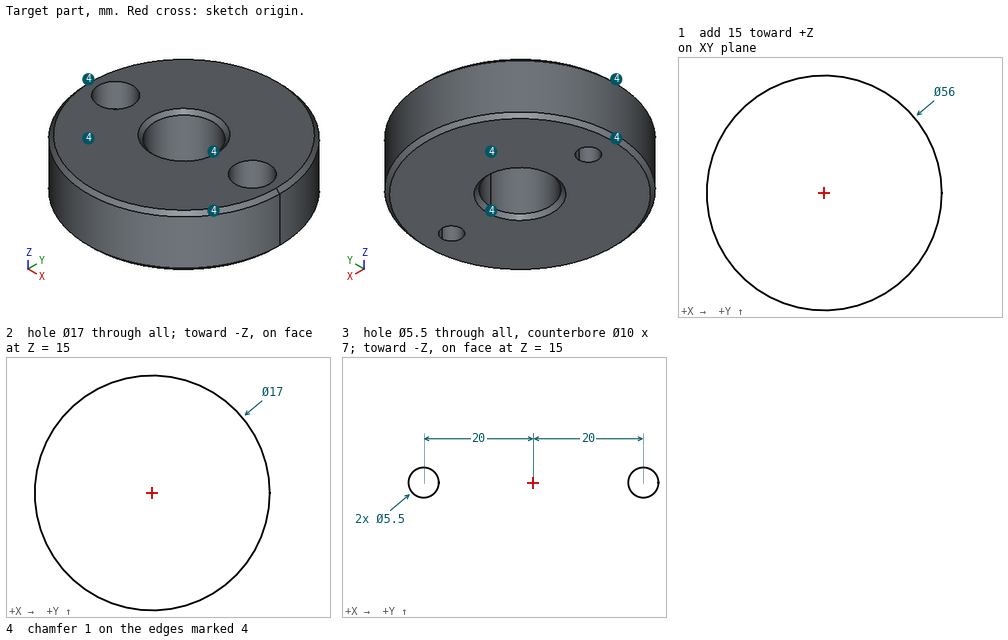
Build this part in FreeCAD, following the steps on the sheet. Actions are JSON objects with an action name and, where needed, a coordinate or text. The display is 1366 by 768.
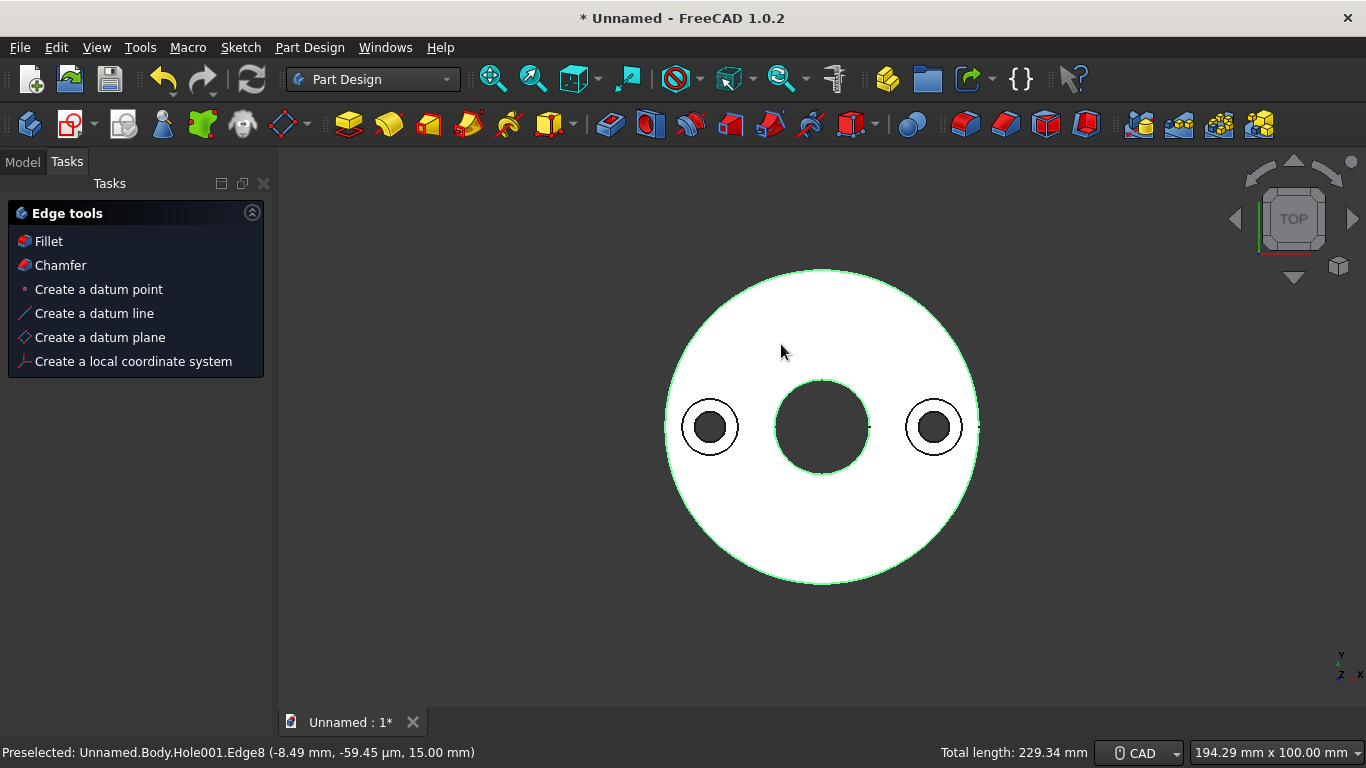
{"action": "key", "text": "1"}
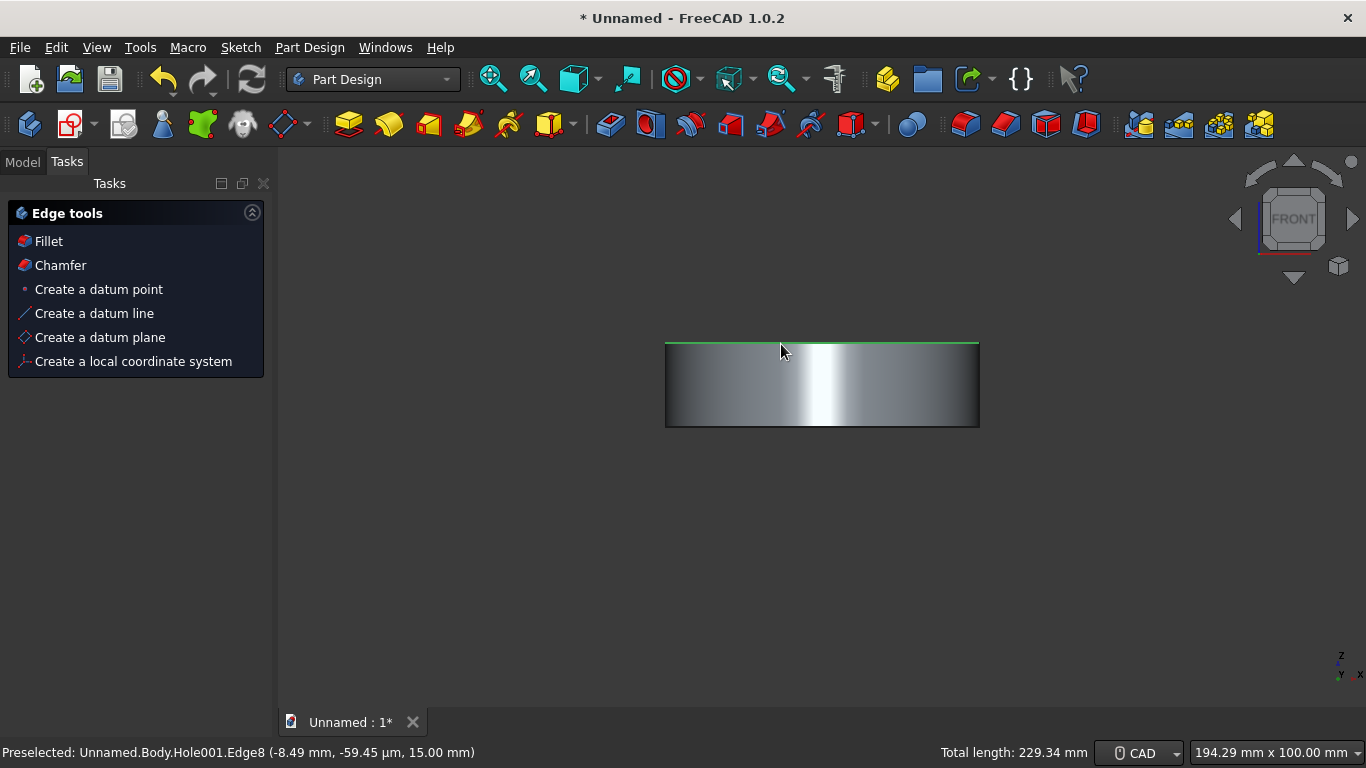
{"action": "left_click", "coordinate": [494, 80]}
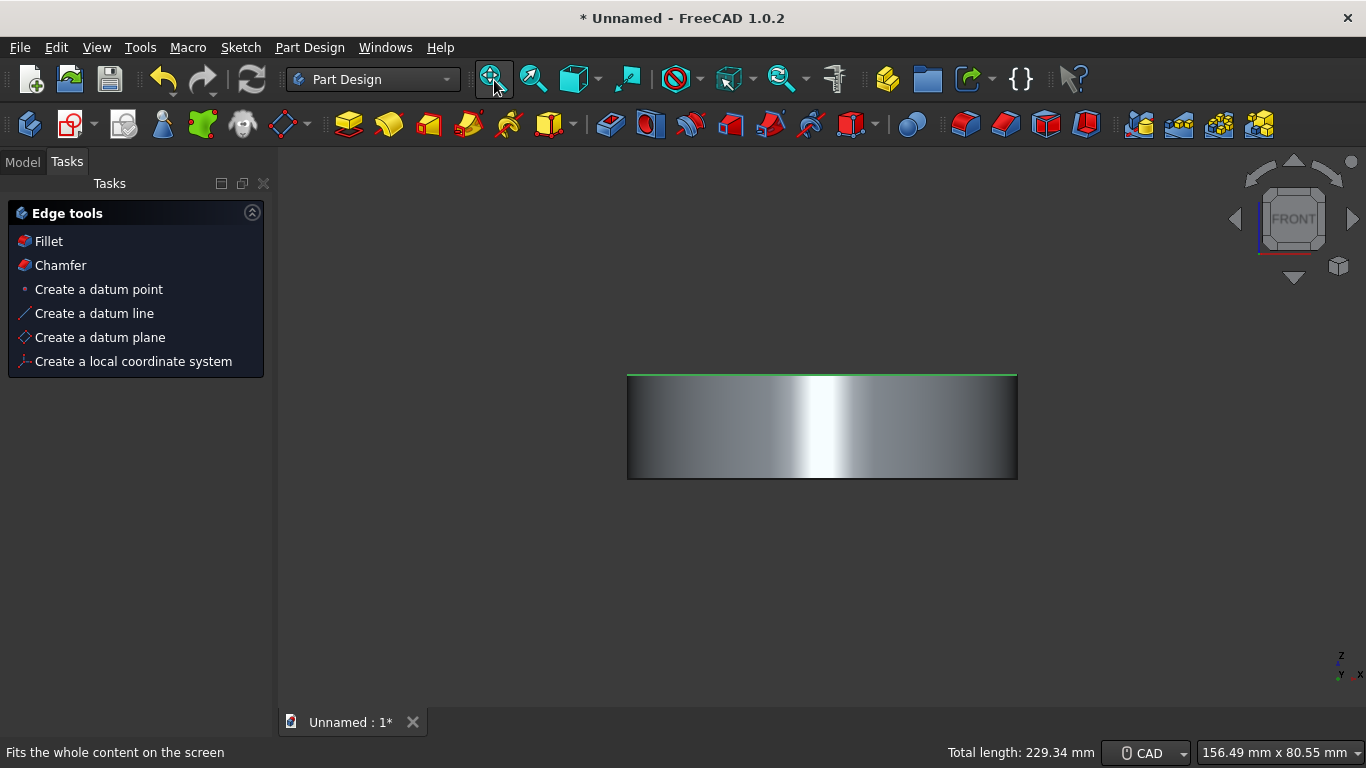
{"action": "left_click", "coordinate": [665, 478], "text": "ctrl"}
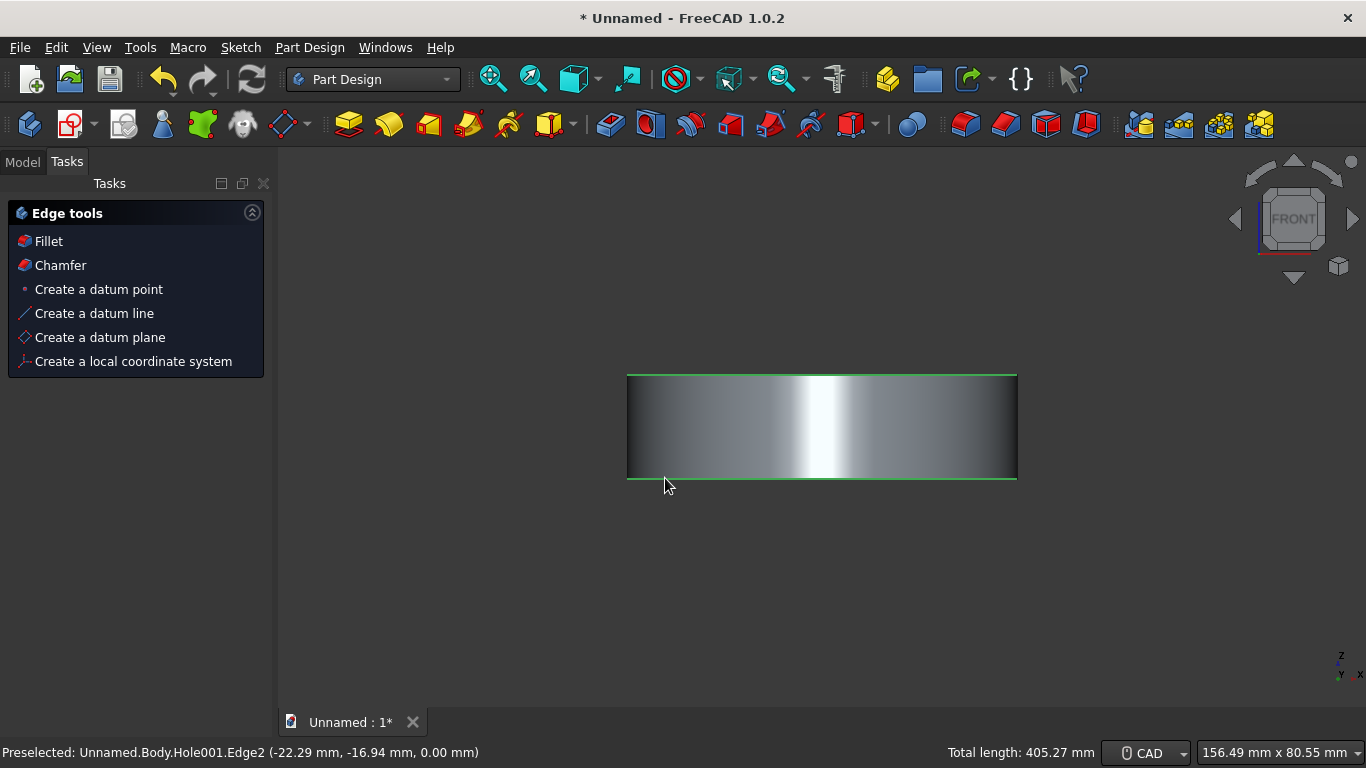
{"action": "key", "text": "3"}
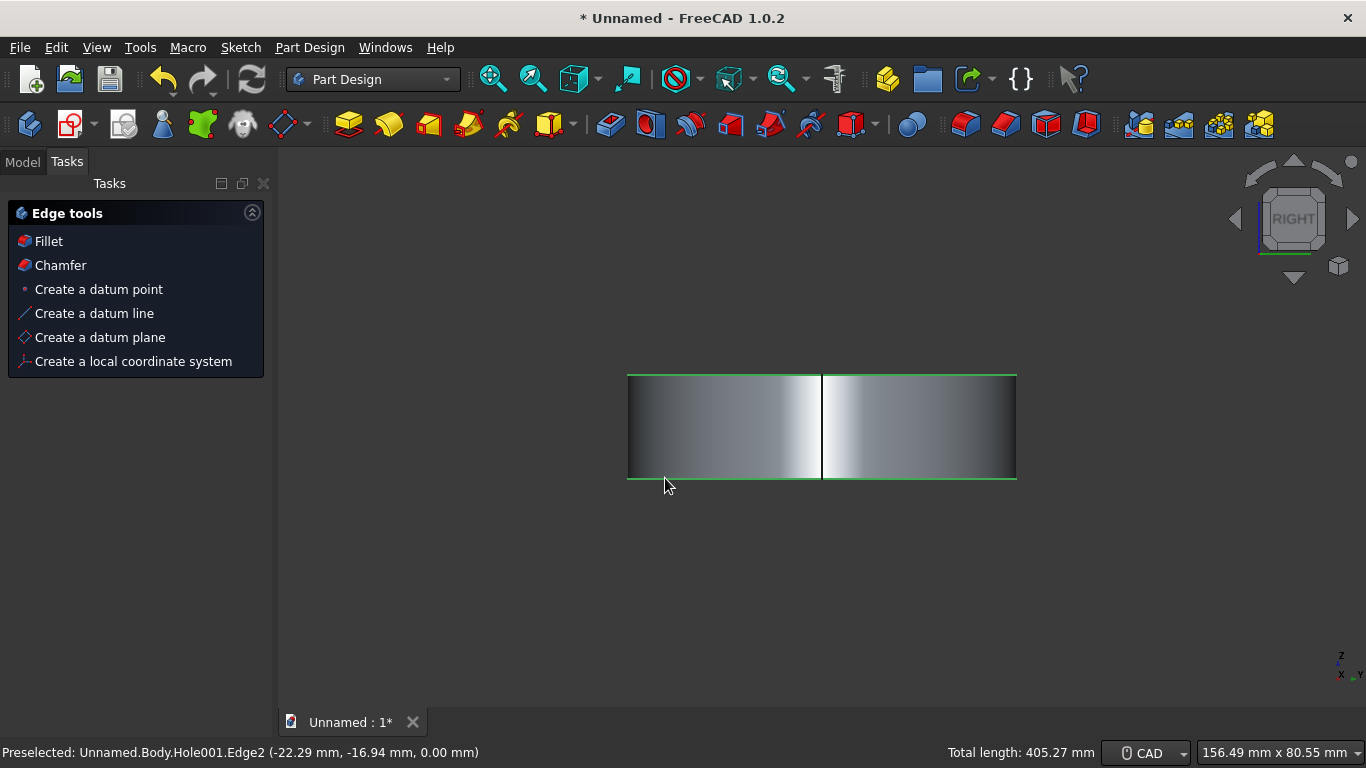
{"action": "left_click", "coordinate": [494, 80]}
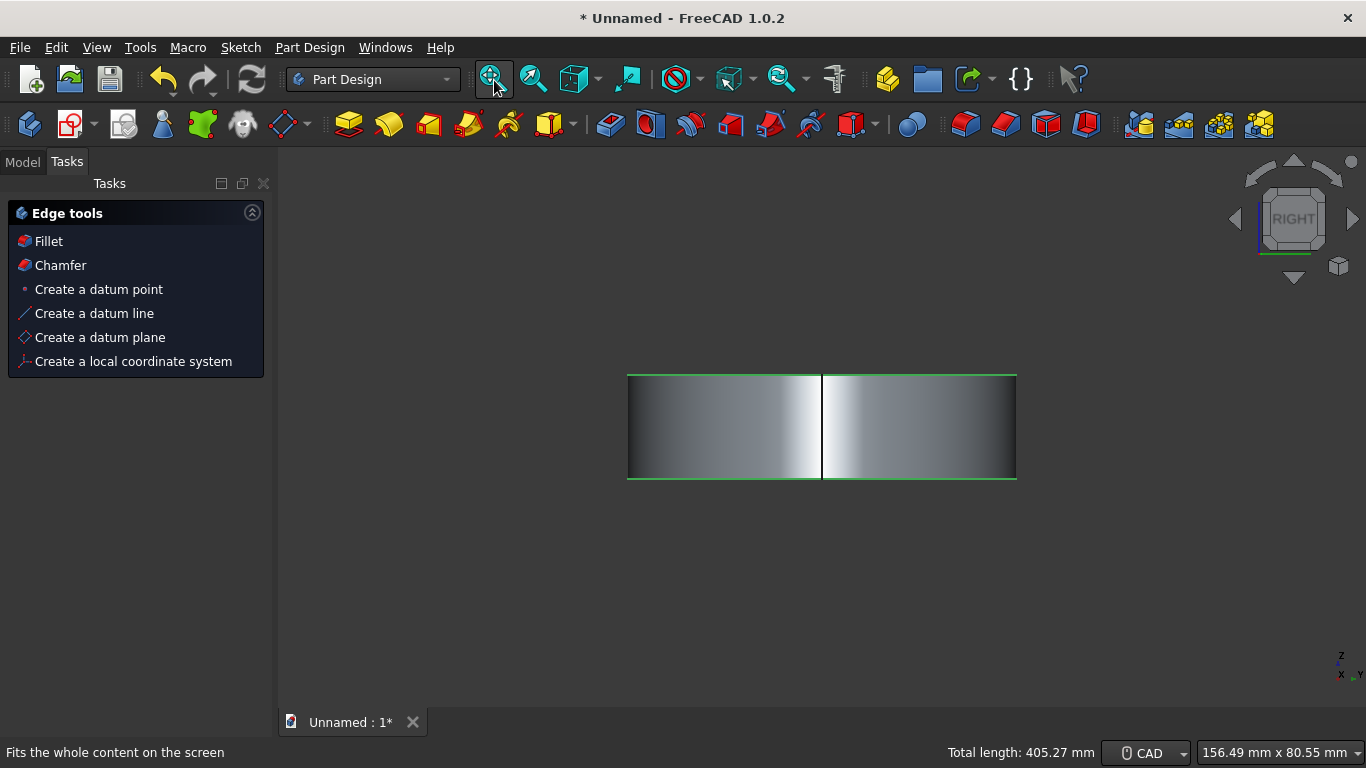
{"action": "key", "text": "5"}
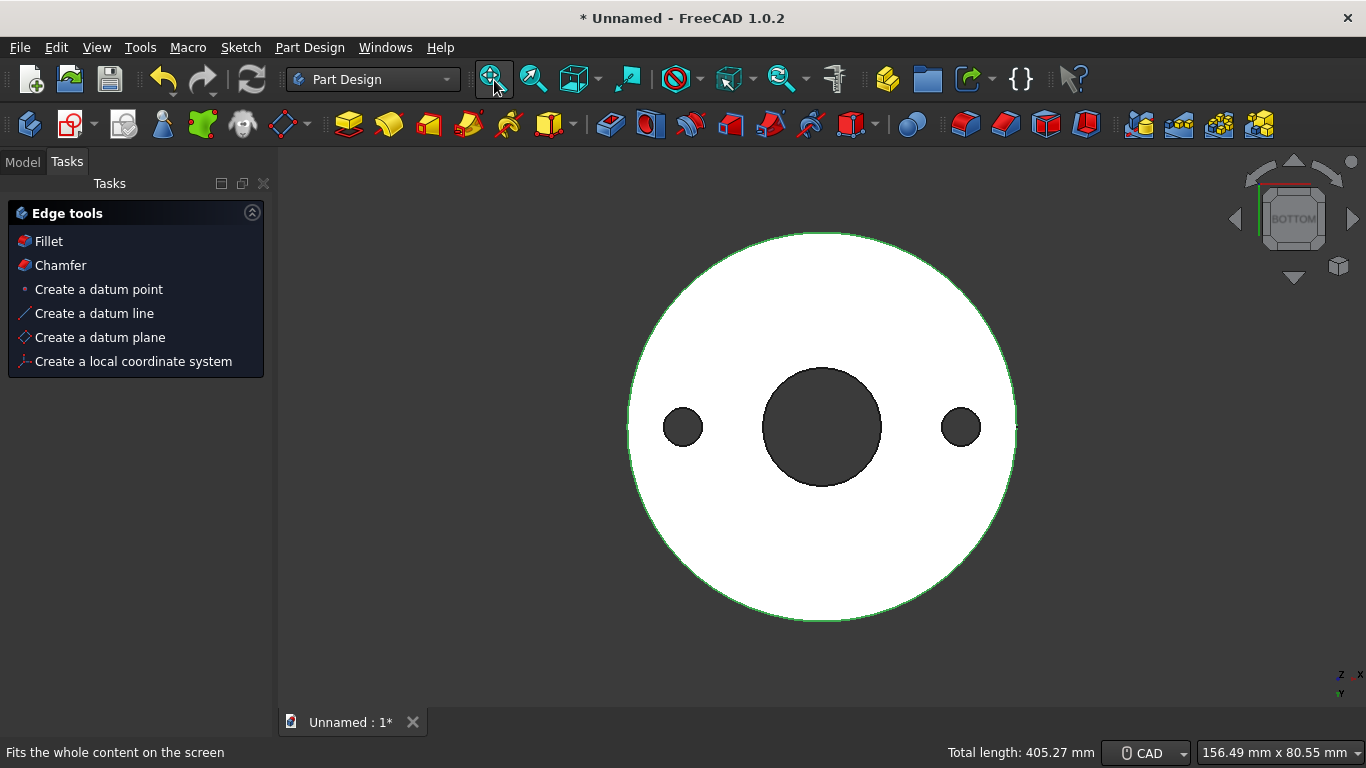
{"action": "left_click", "coordinate": [763, 426], "text": "ctrl"}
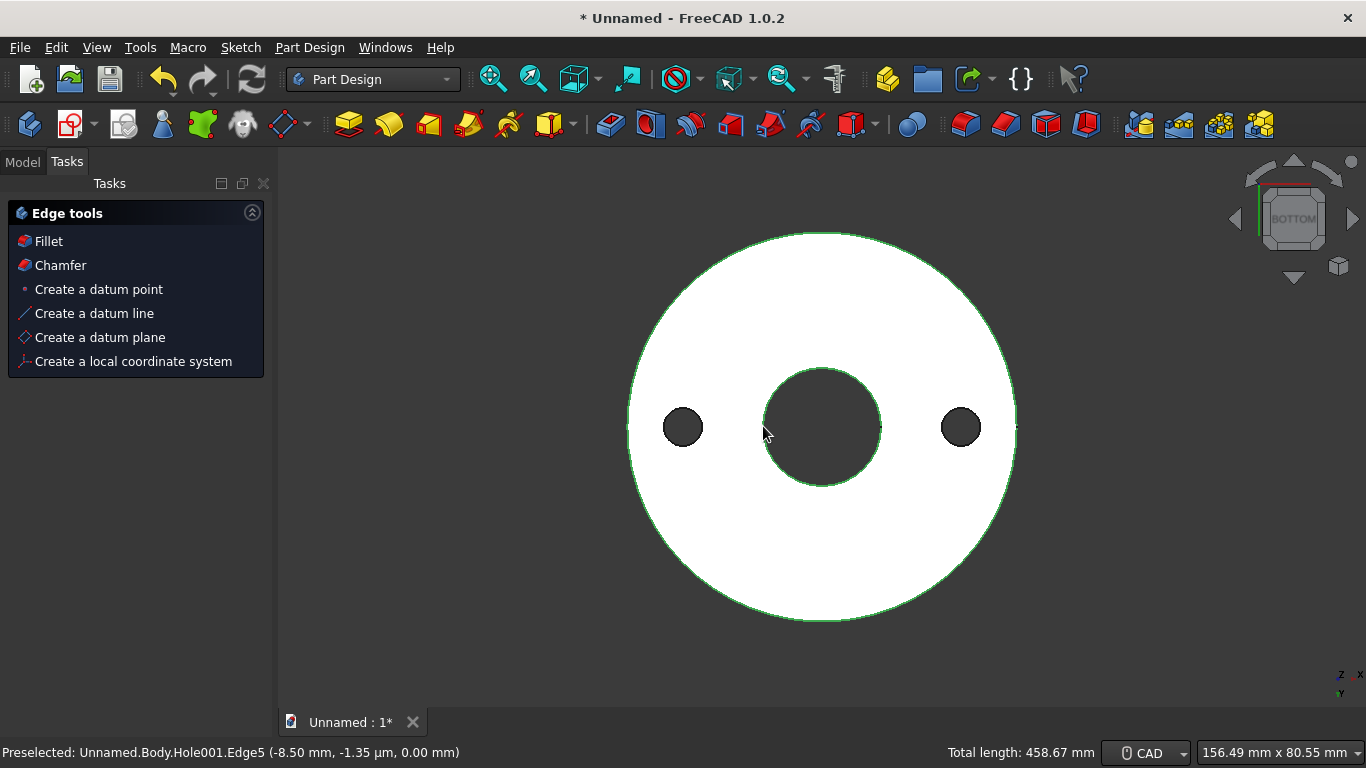
{"action": "left_click", "coordinate": [1006, 124]}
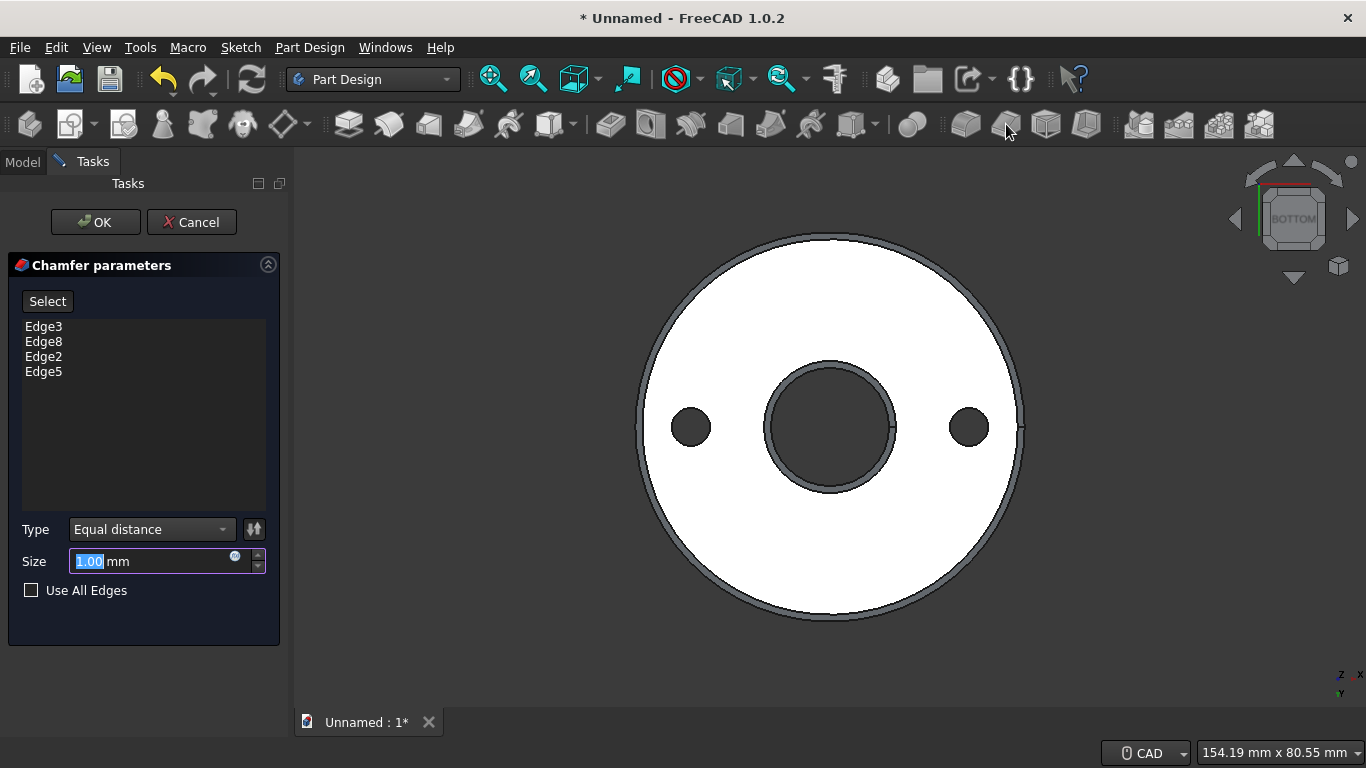
{"action": "type", "text": "1"}
{"action": "key", "text": "Tab"}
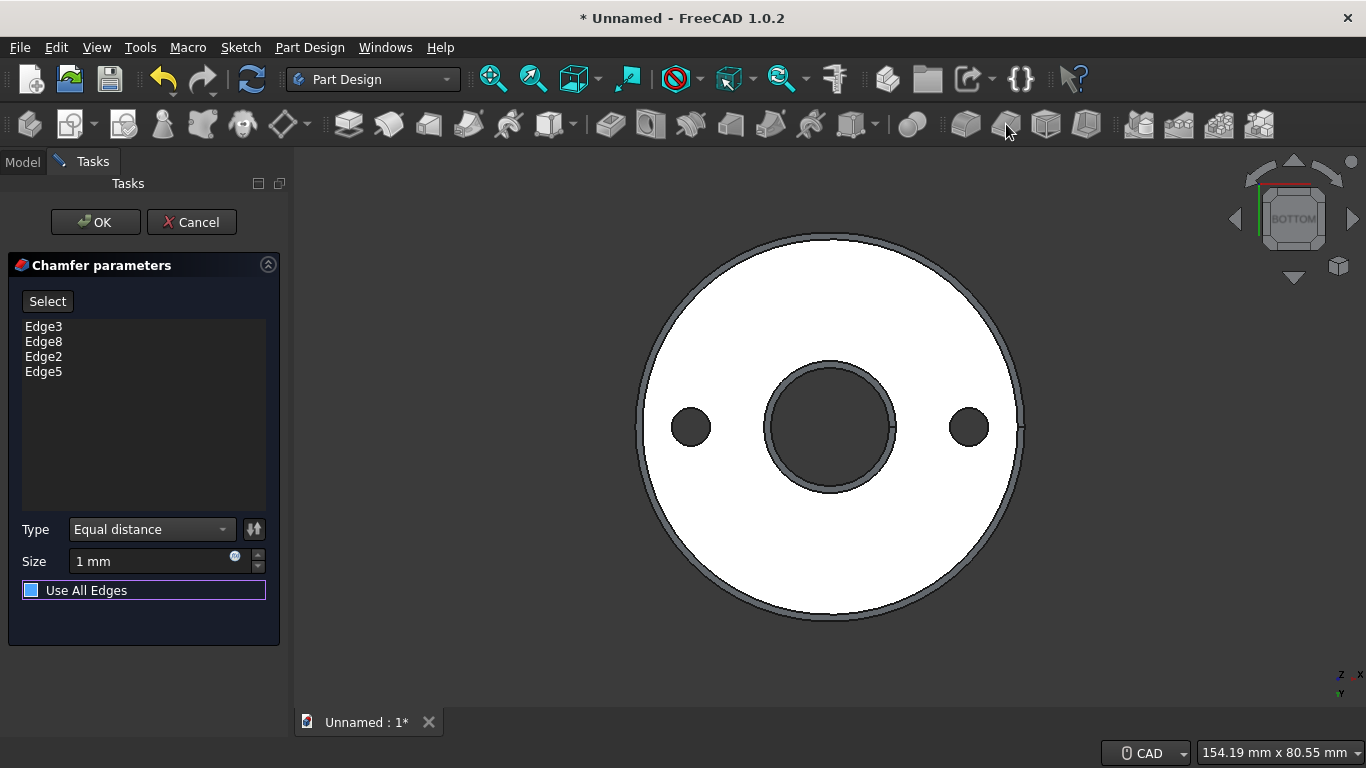
{"action": "left_click", "coordinate": [96, 222]}